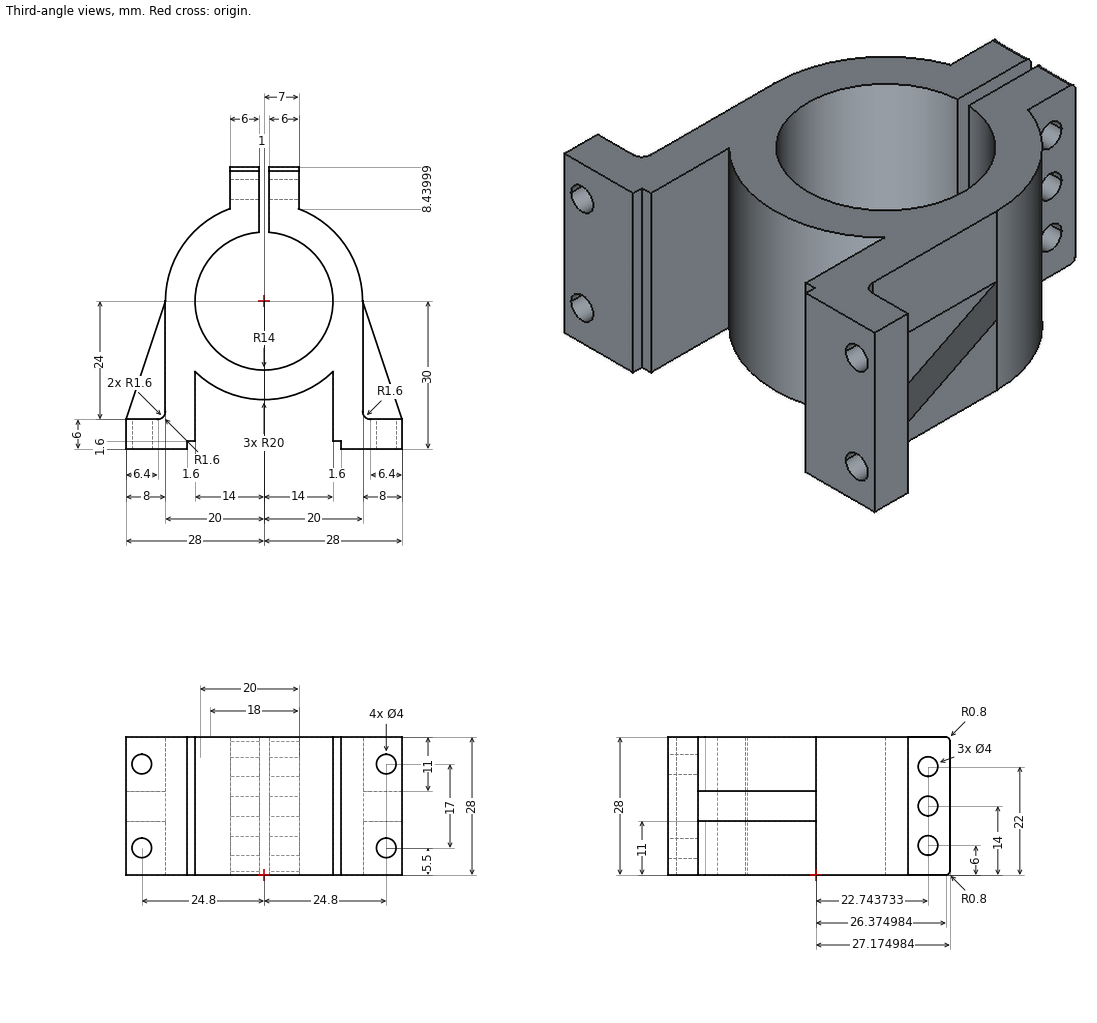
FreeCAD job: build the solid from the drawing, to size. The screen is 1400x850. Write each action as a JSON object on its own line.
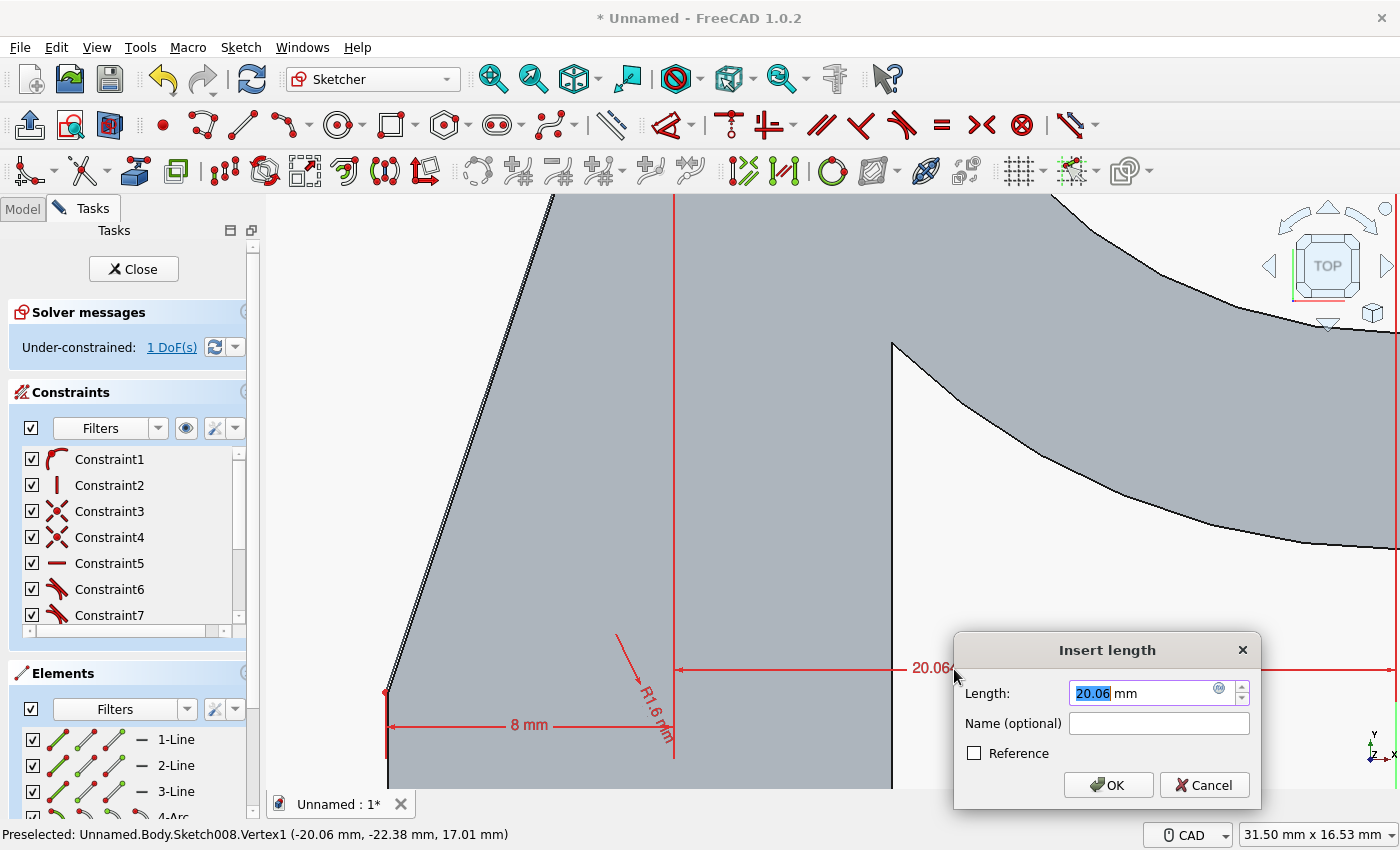
{"action": "type", "text": "20"}
{"action": "key", "text": "Return"}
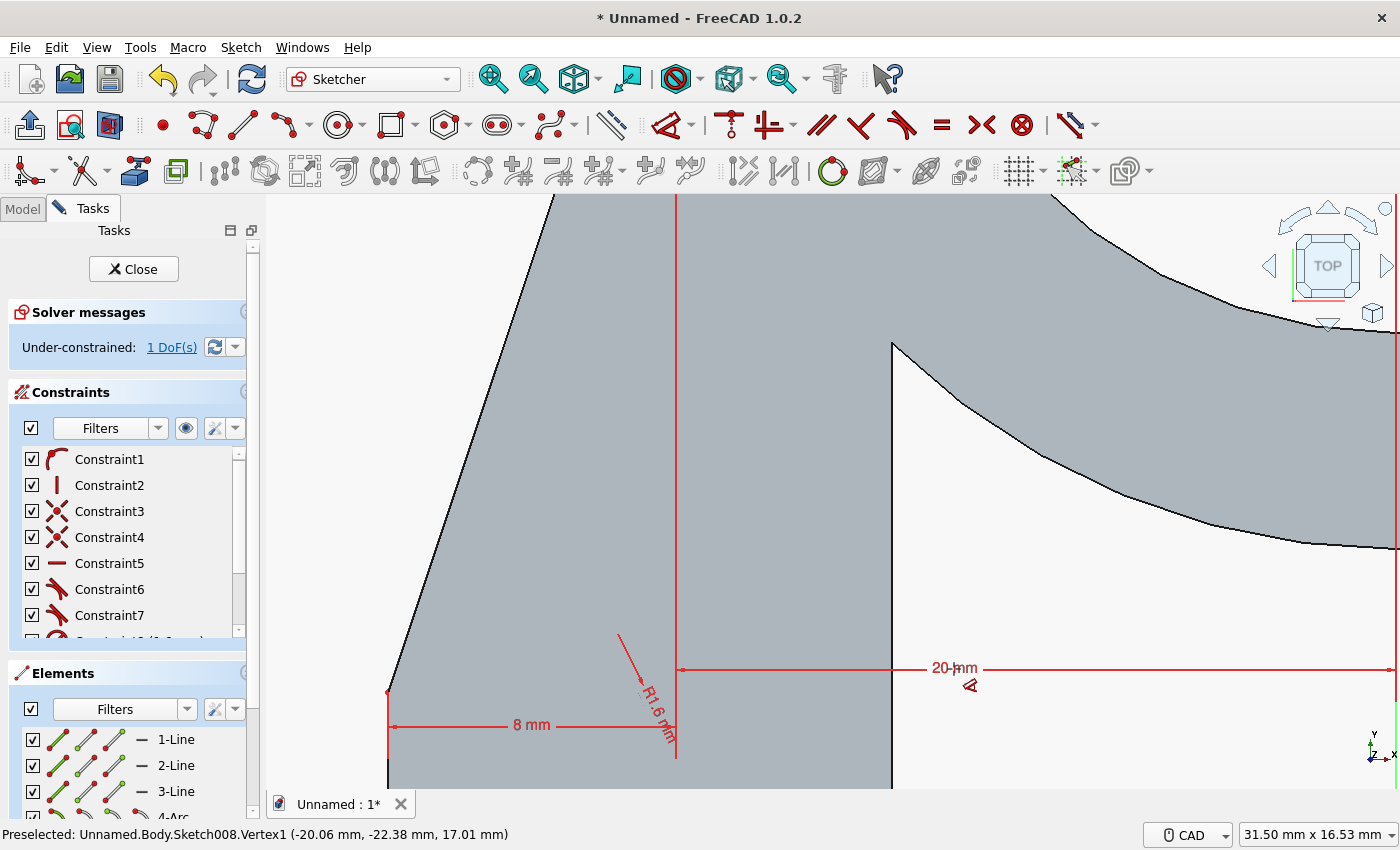
{"action": "left_click", "coordinate": [388, 692]}
{"action": "left_click", "coordinate": [354, 457]}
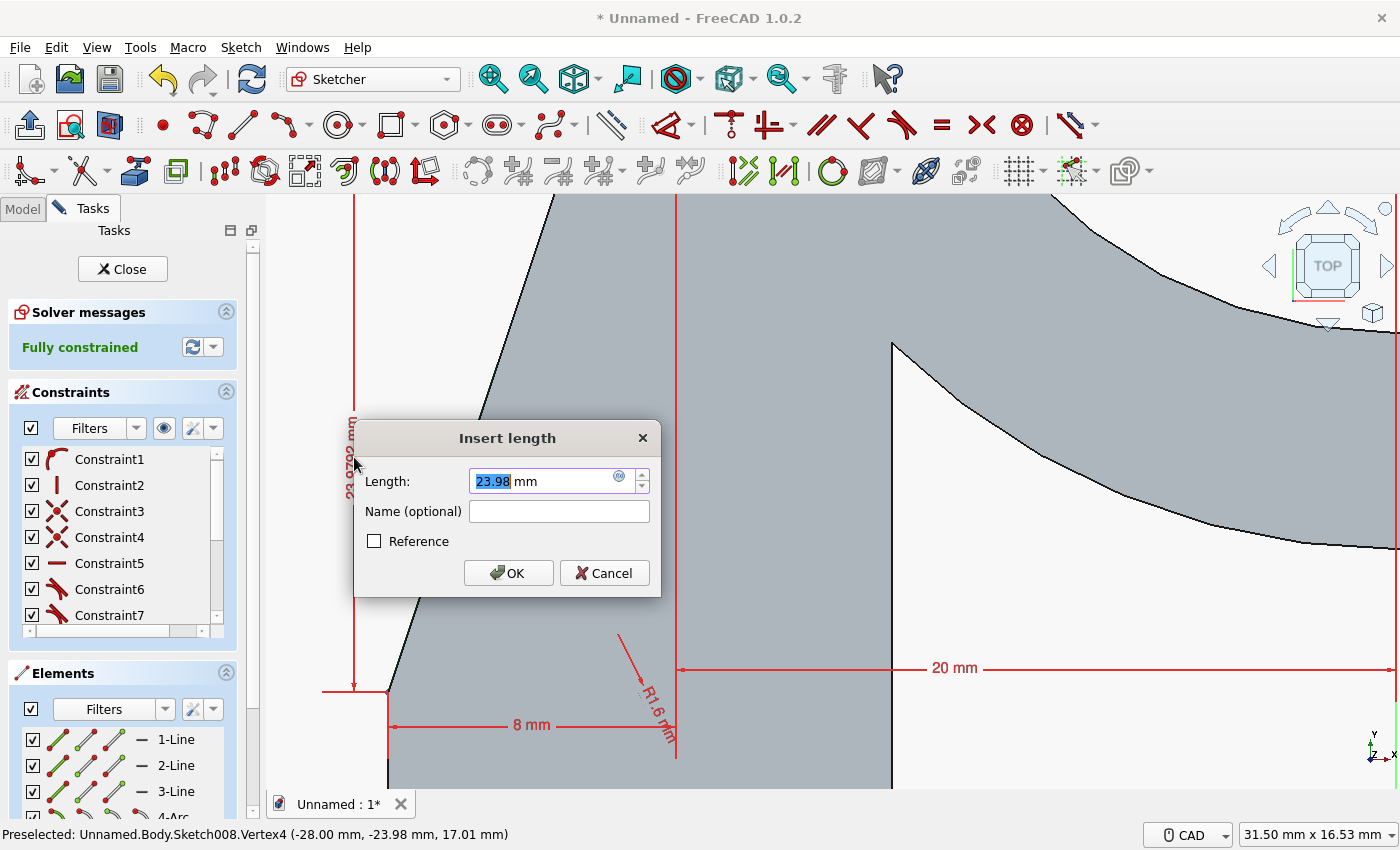
{"action": "type", "text": "24"}
{"action": "key", "text": "Return"}
{"action": "key", "text": "Escape"}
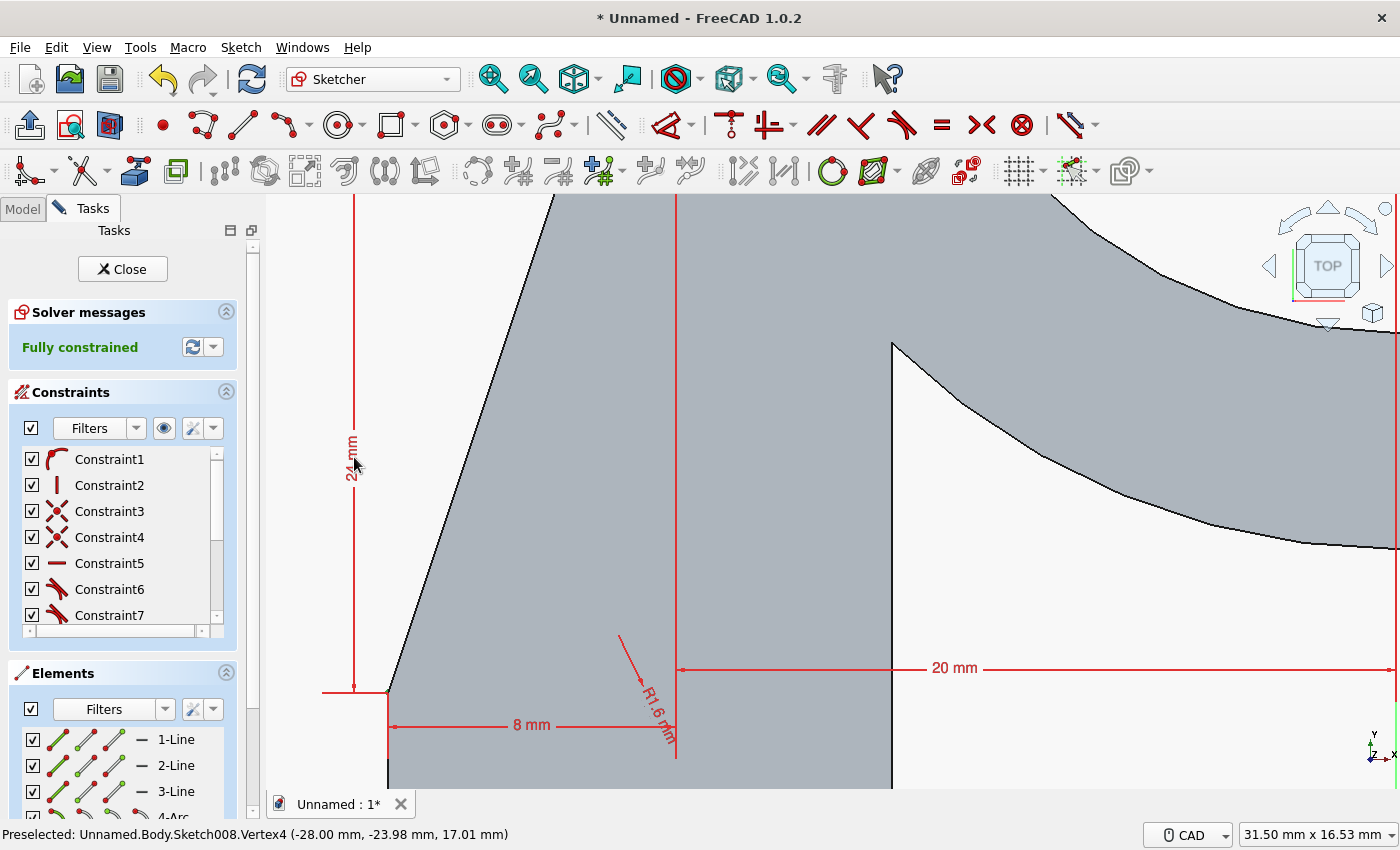
{"action": "left_click", "coordinate": [123, 269]}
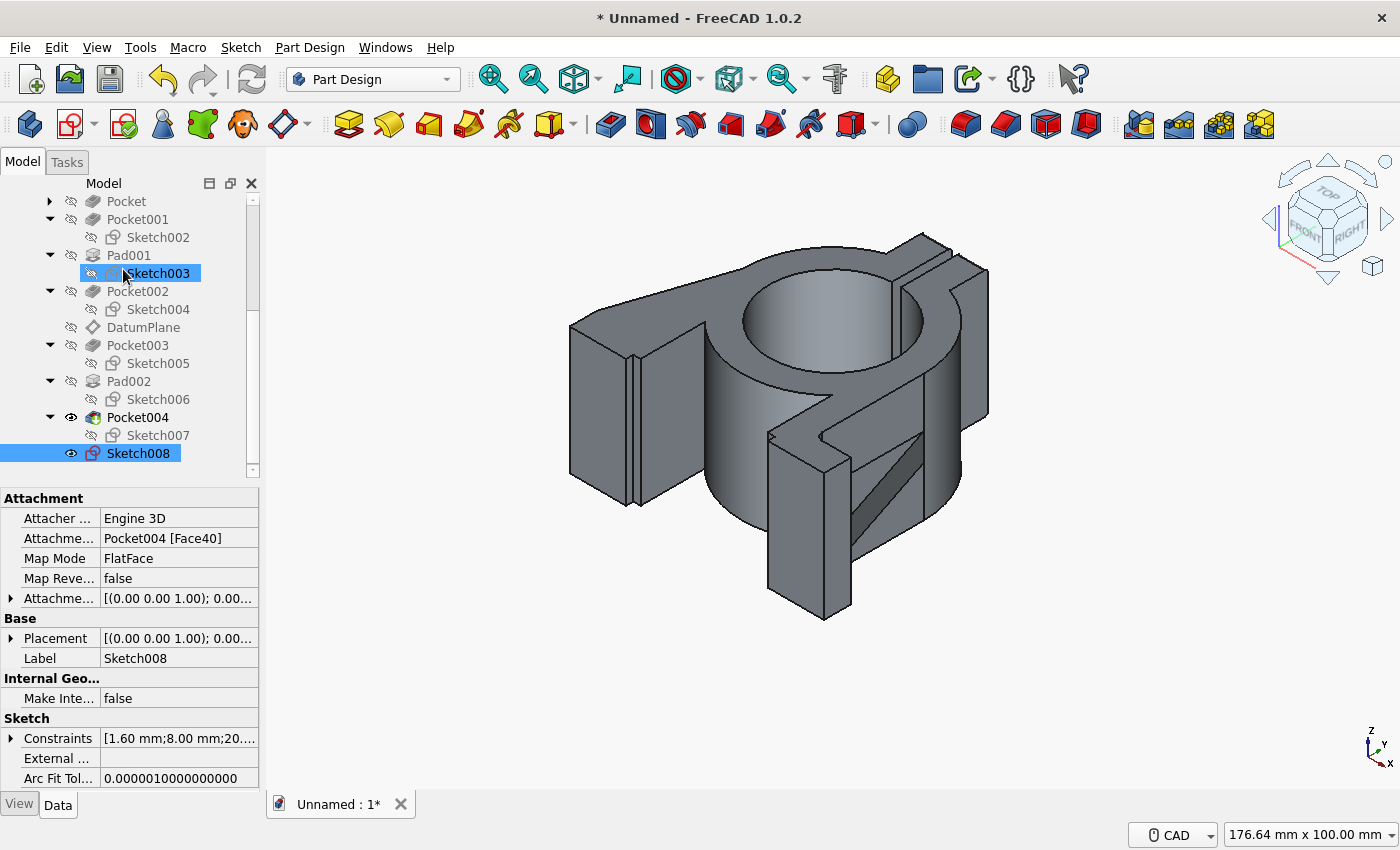
{"action": "left_click", "coordinate": [612, 124]}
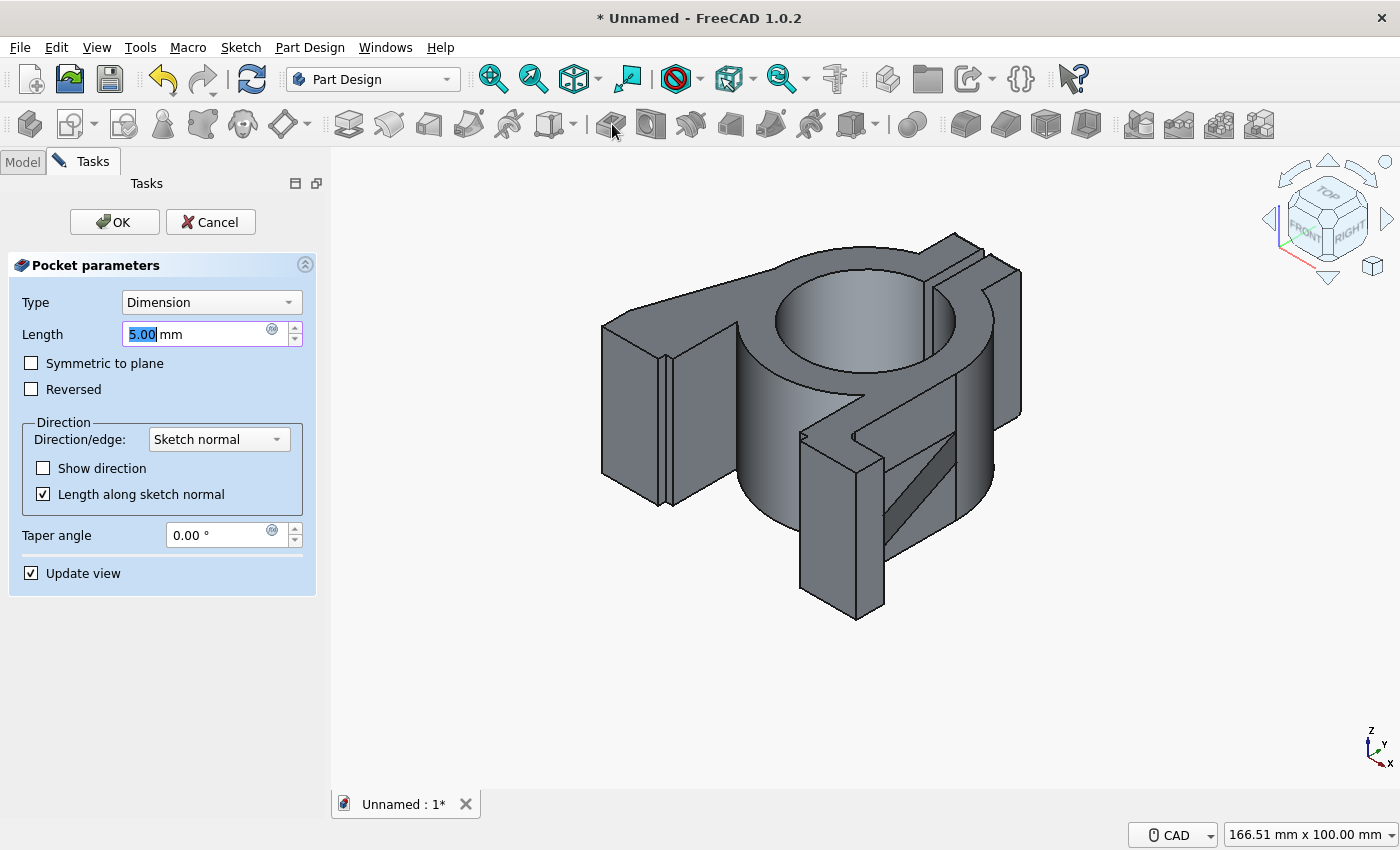
{"action": "type", "text": "11"}
{"action": "key", "text": "Tab"}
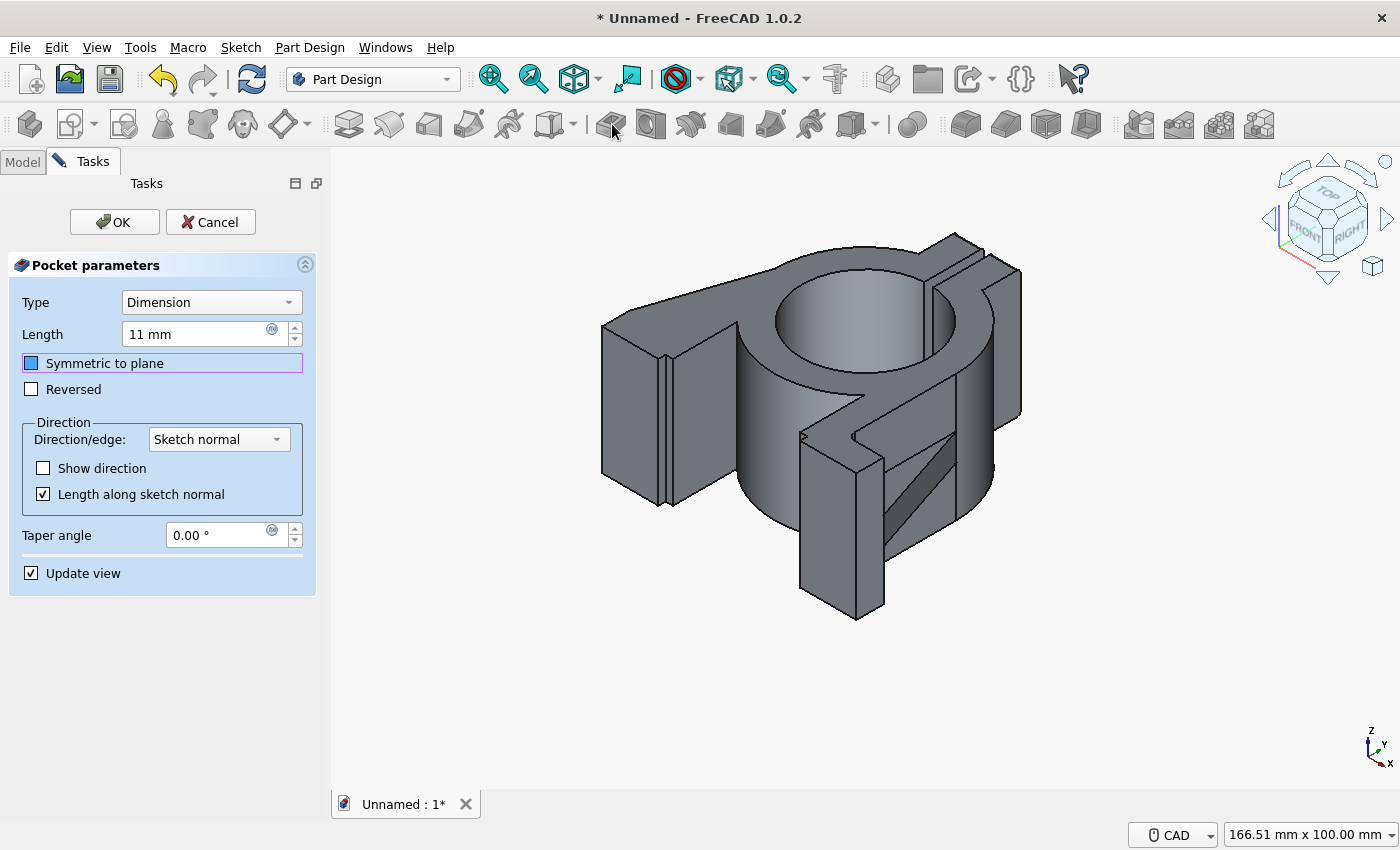
{"action": "left_click", "coordinate": [30, 389]}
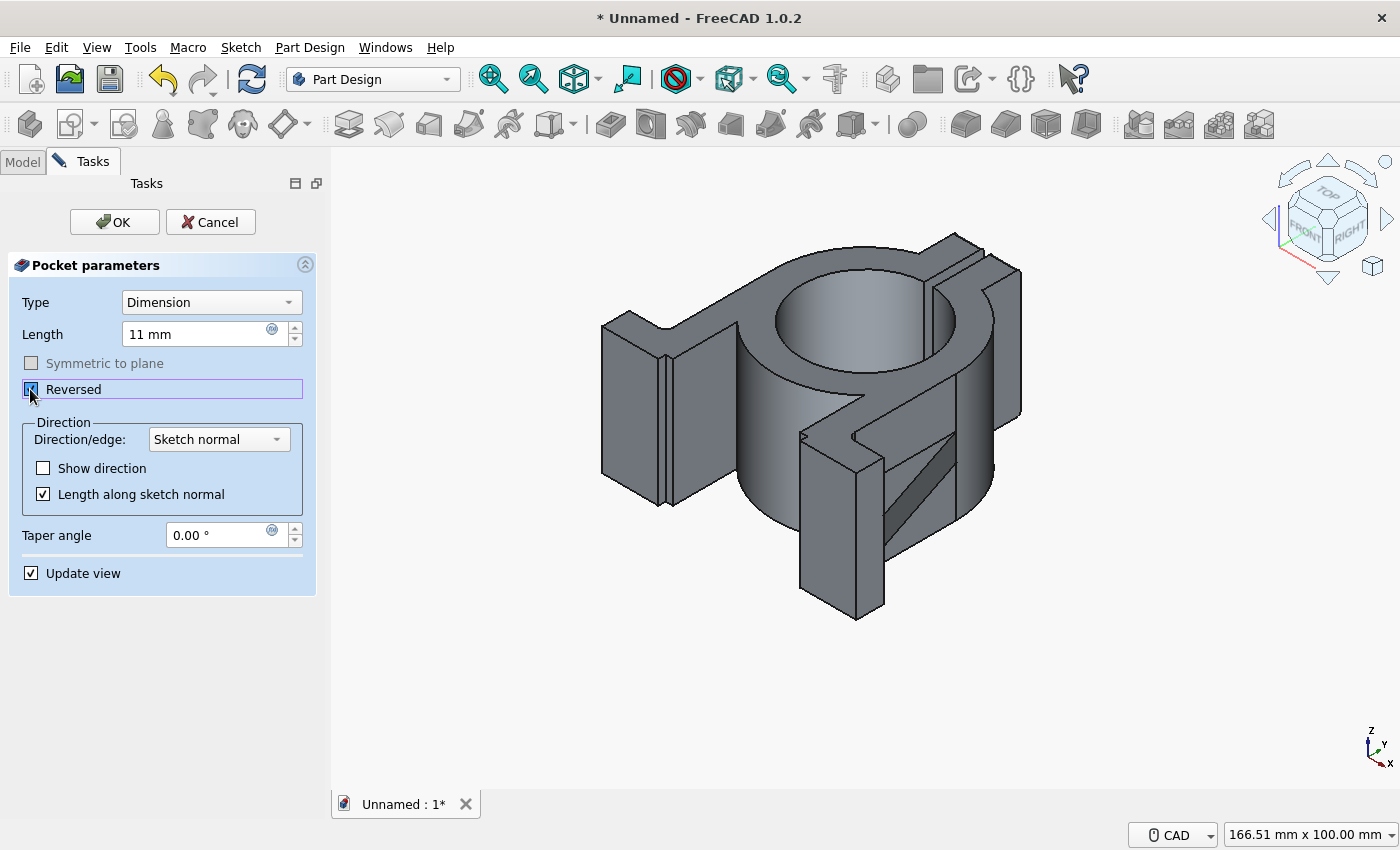
{"action": "left_click", "coordinate": [115, 222]}